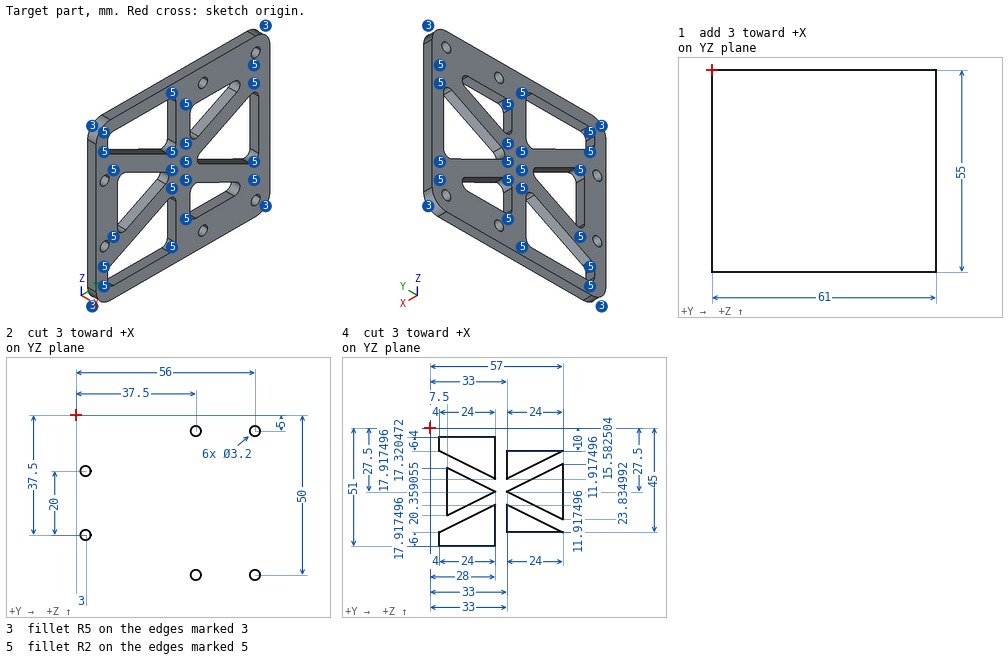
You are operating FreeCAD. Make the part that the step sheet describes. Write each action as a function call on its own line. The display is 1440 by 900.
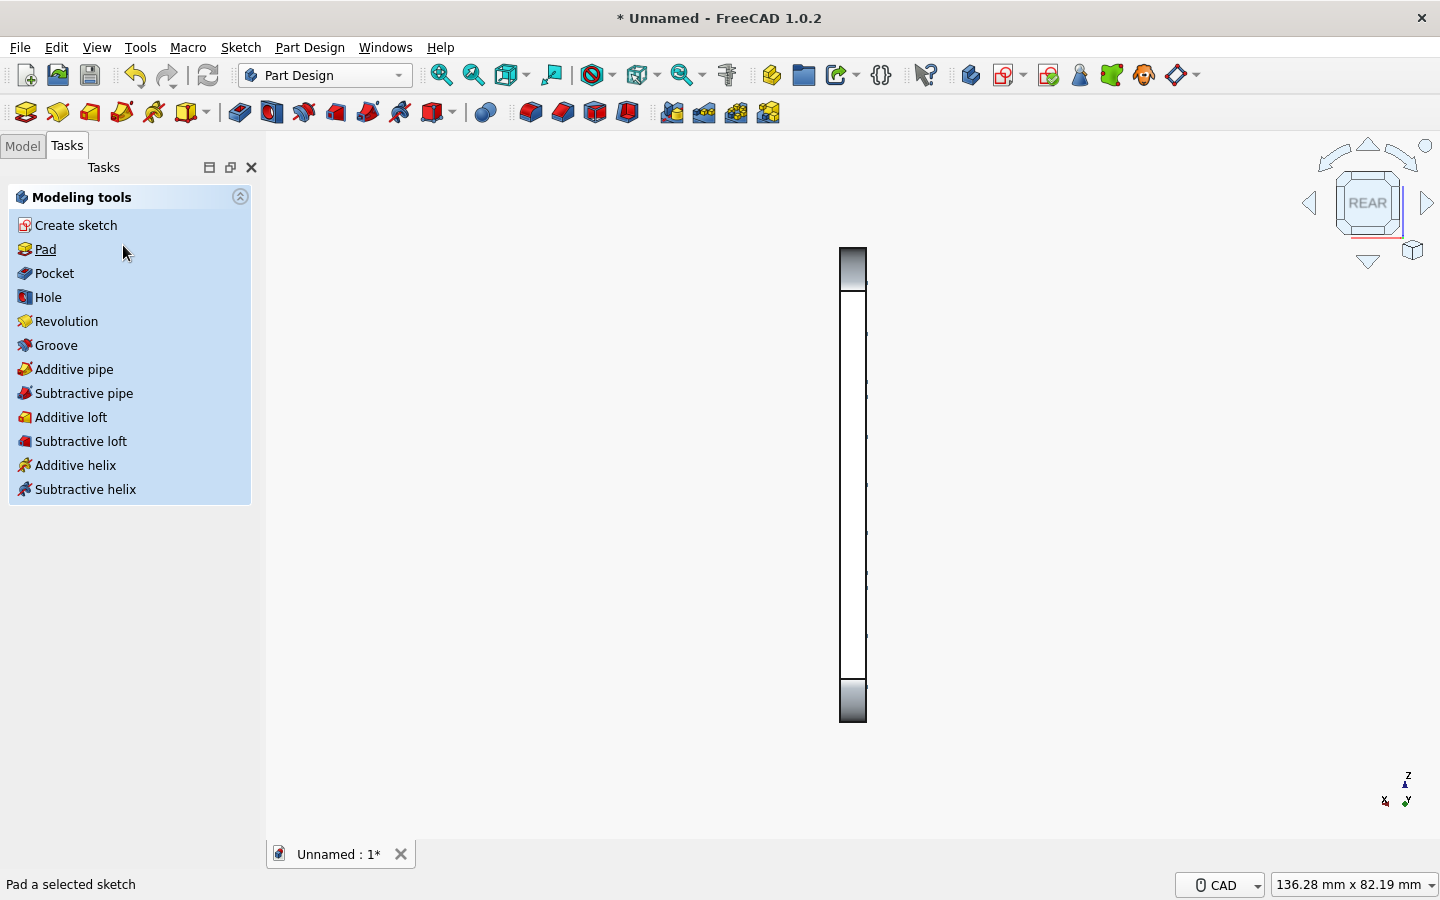
click(240, 112)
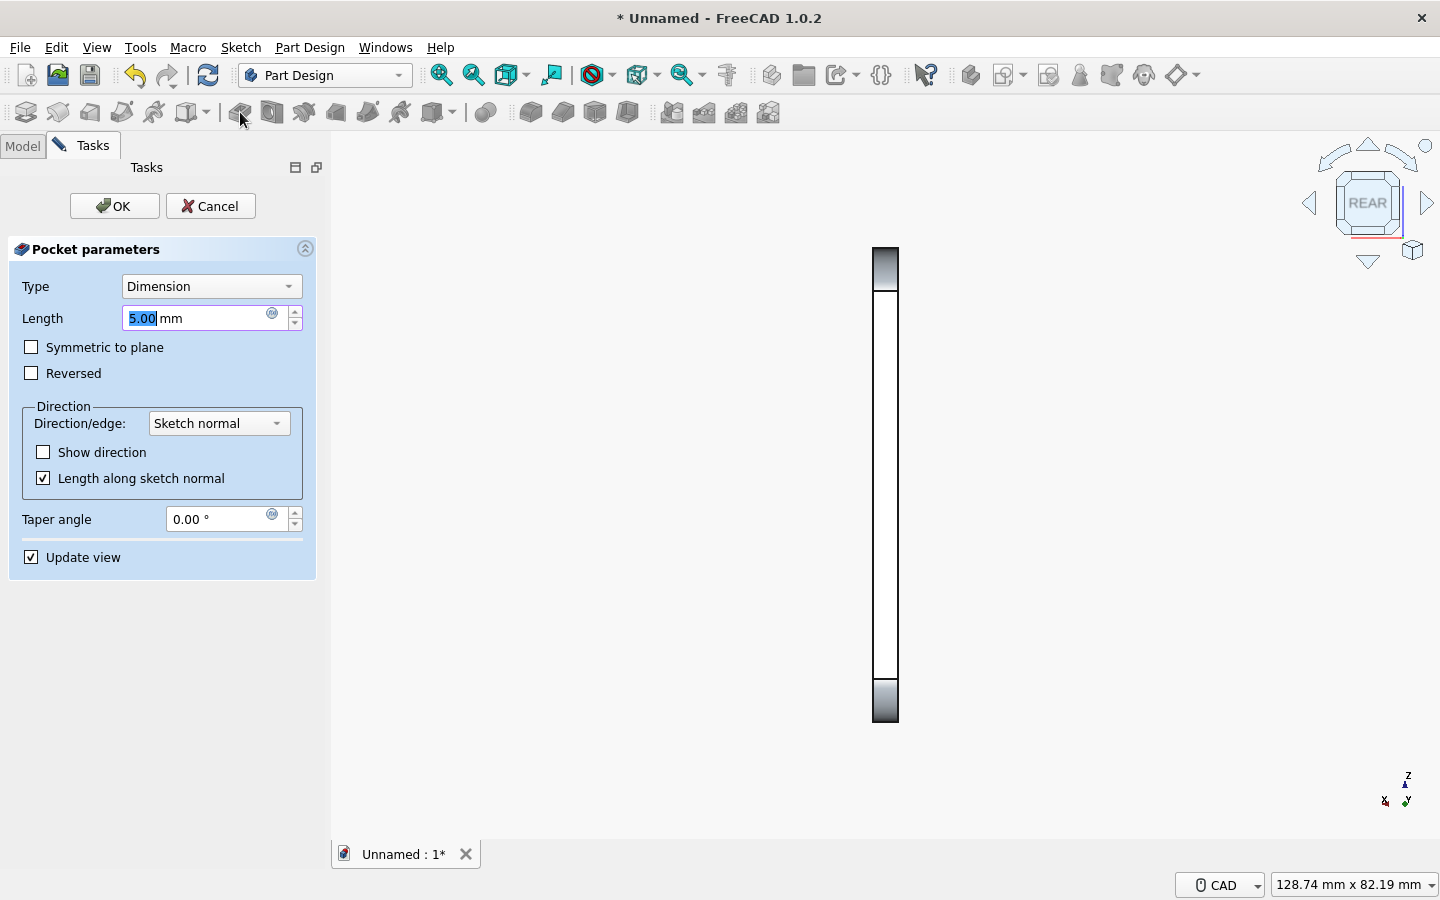
text(3)
key(Tab)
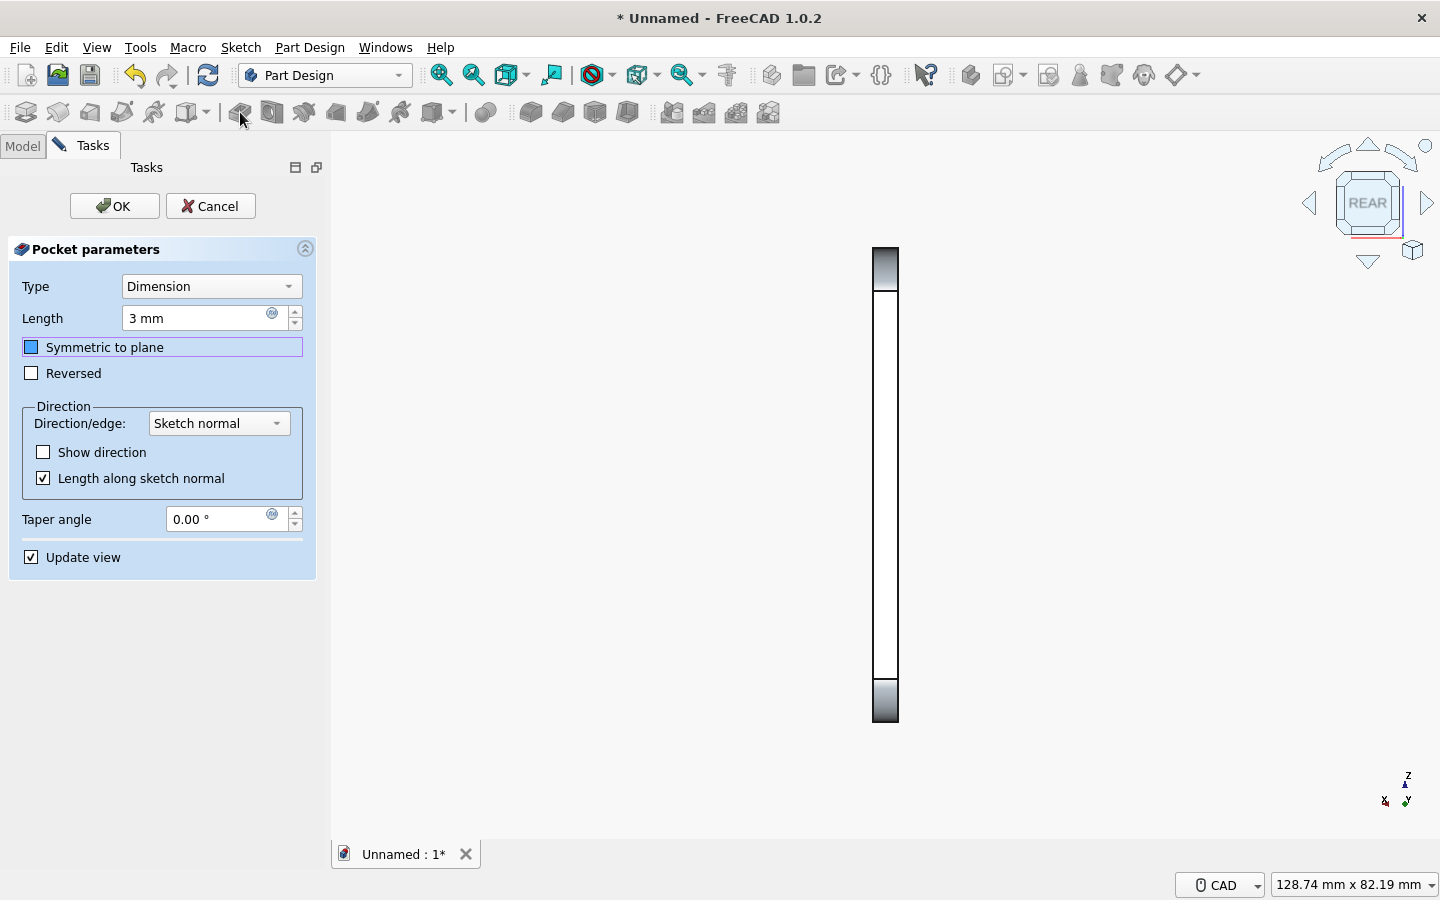
click(30, 373)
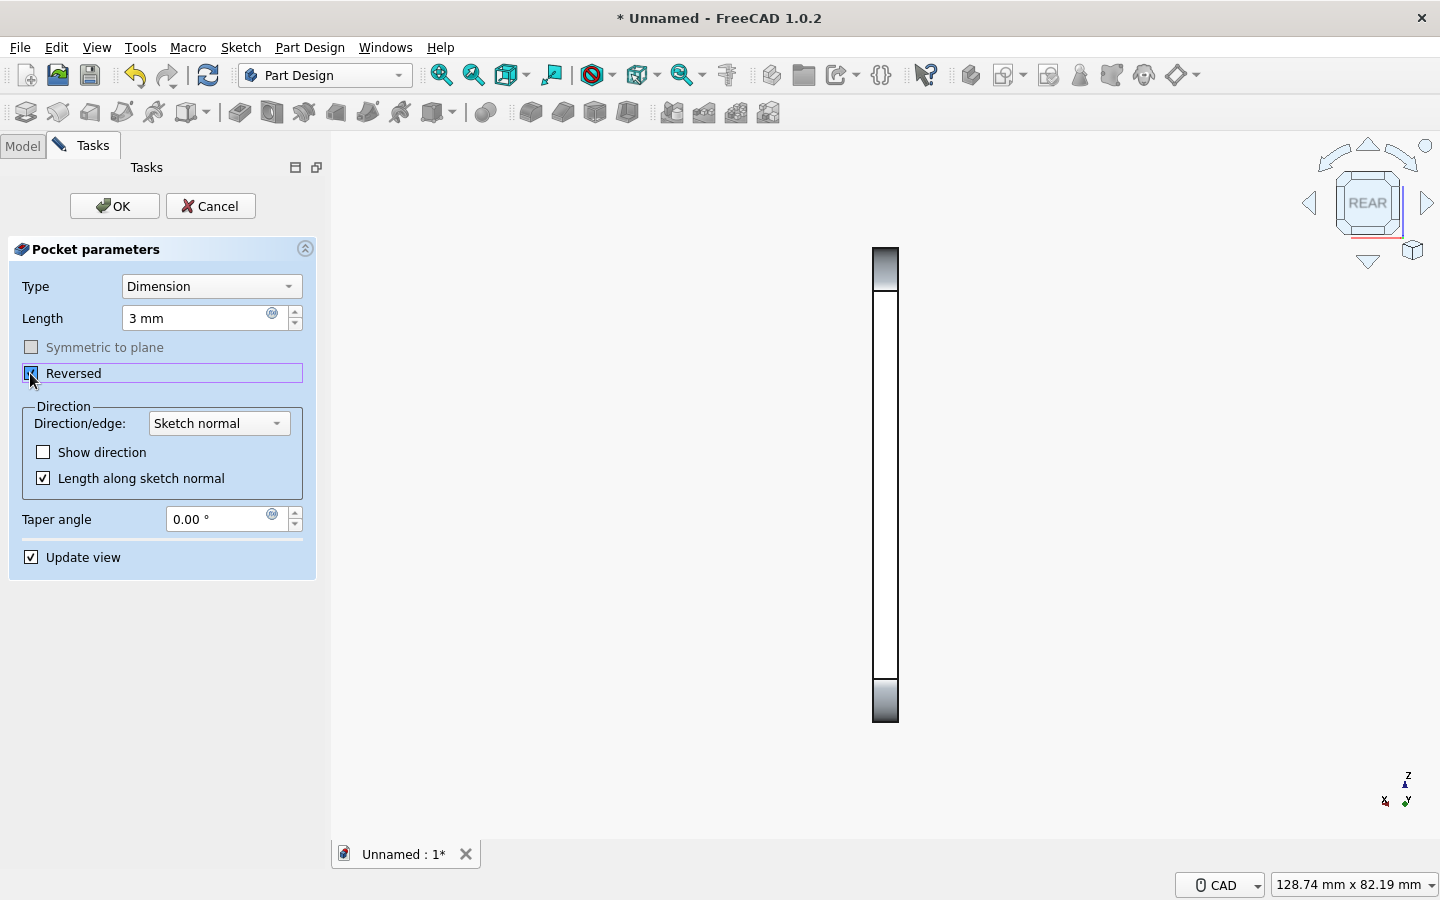
click(115, 206)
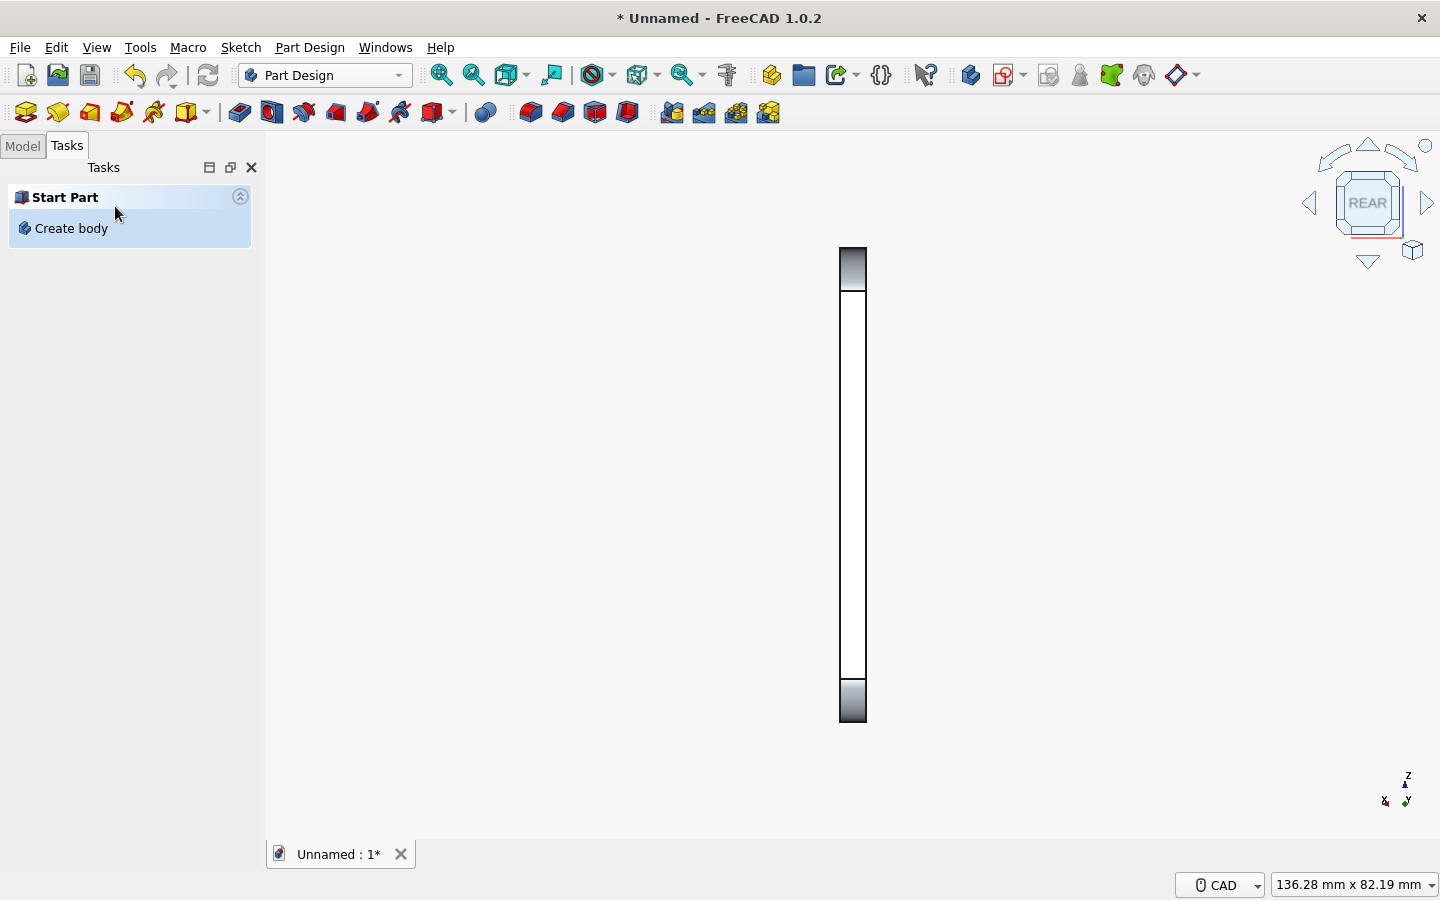
key(0)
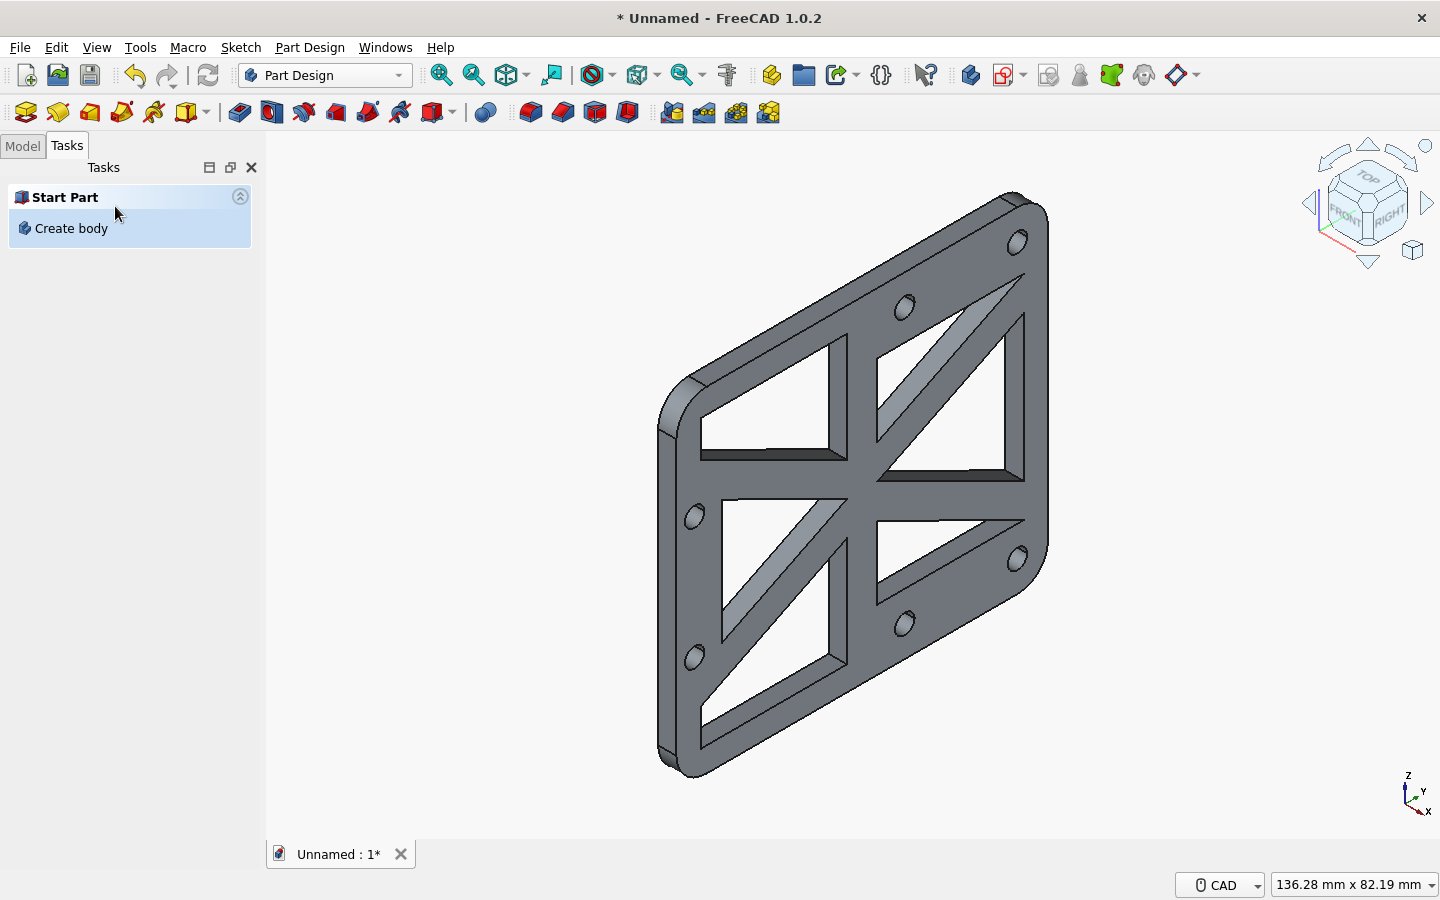
key(2)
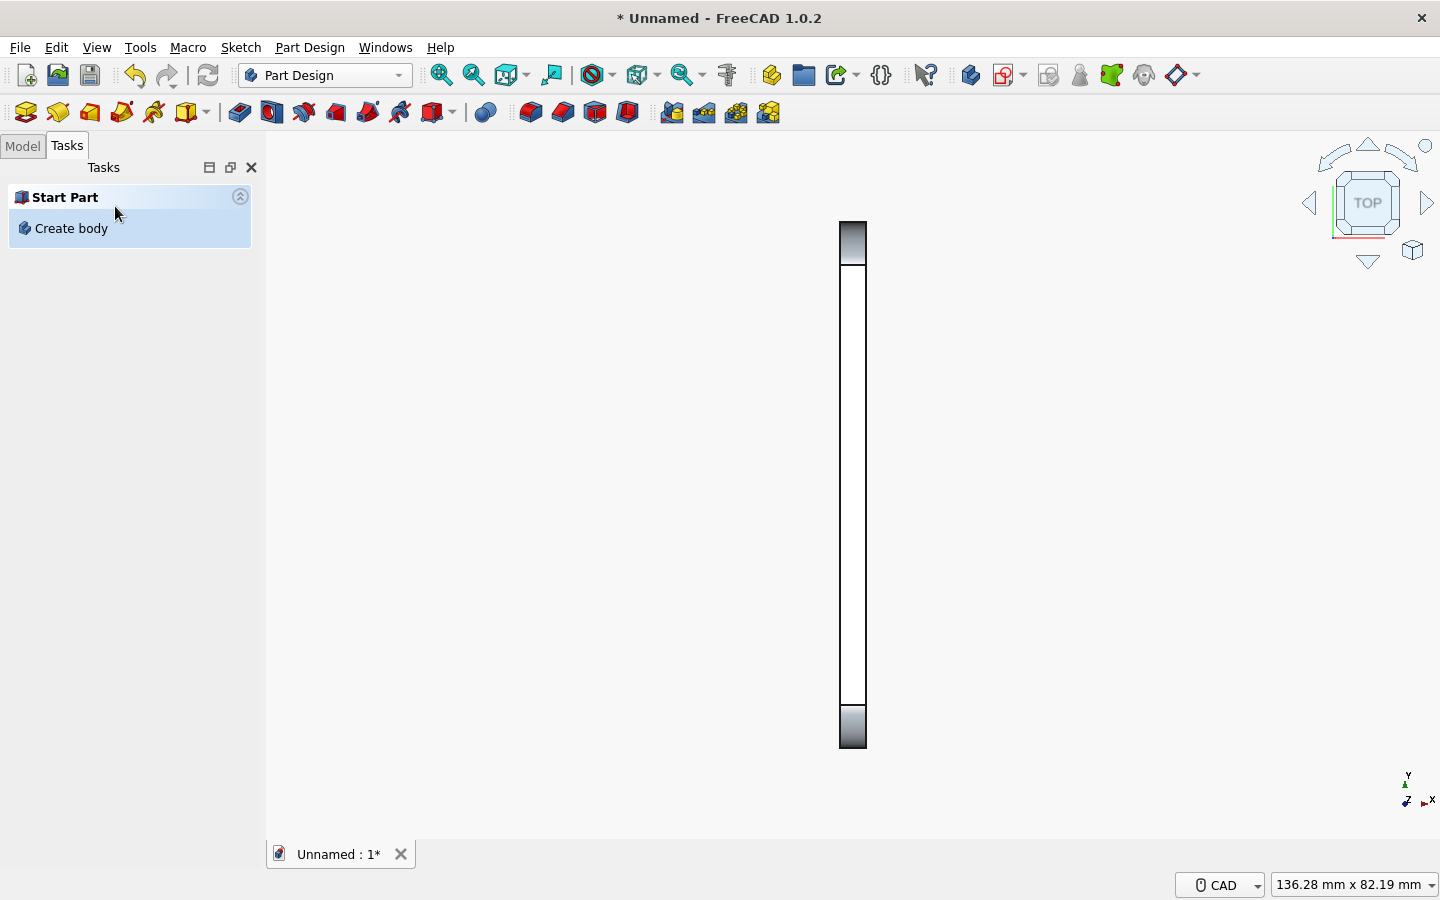
key(1)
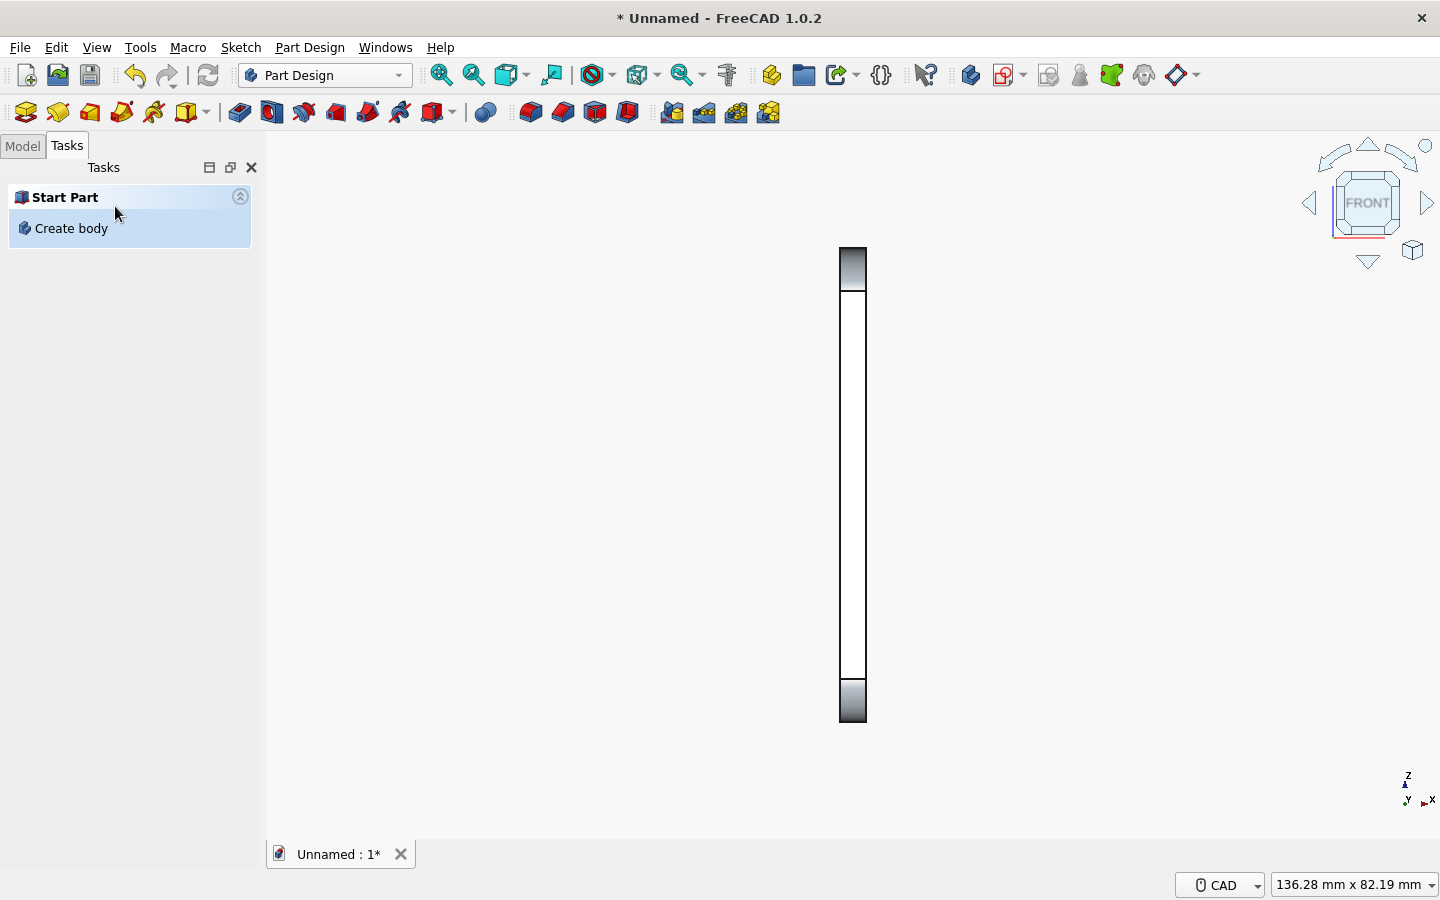
key(3)